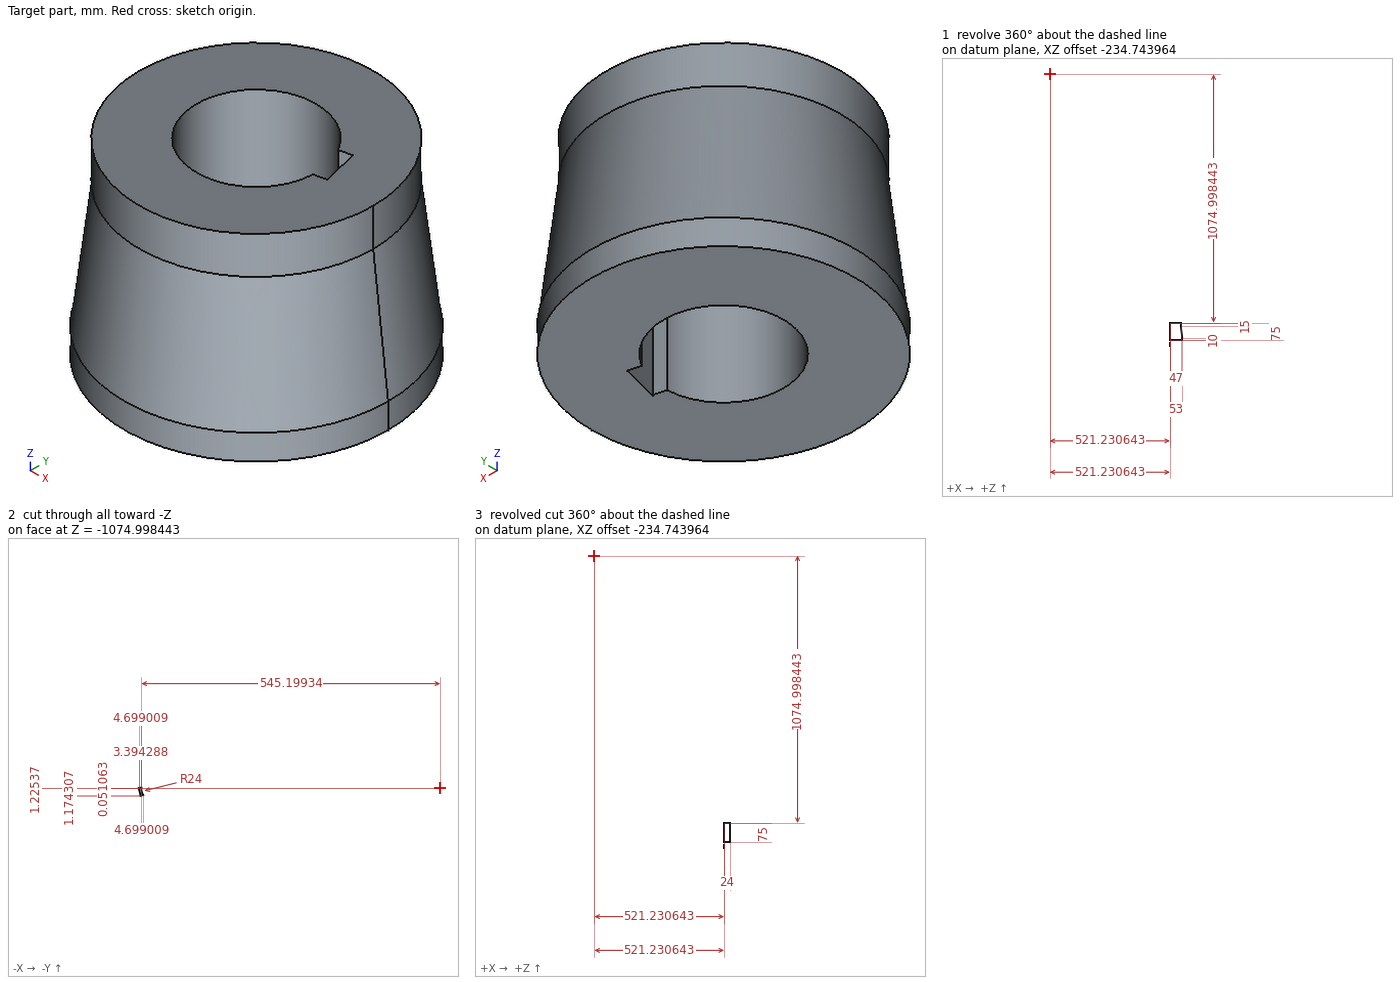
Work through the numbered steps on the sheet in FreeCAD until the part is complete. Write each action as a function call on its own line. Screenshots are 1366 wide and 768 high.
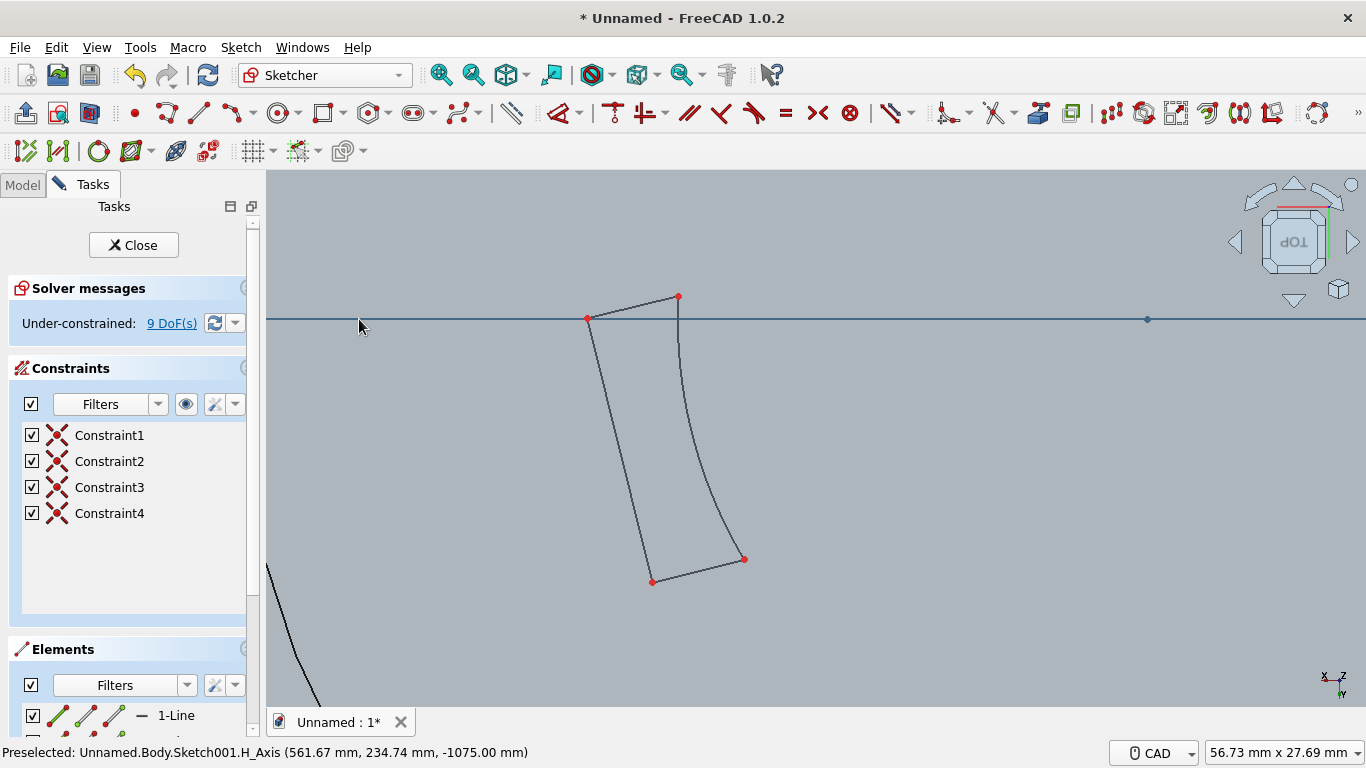
click(614, 114)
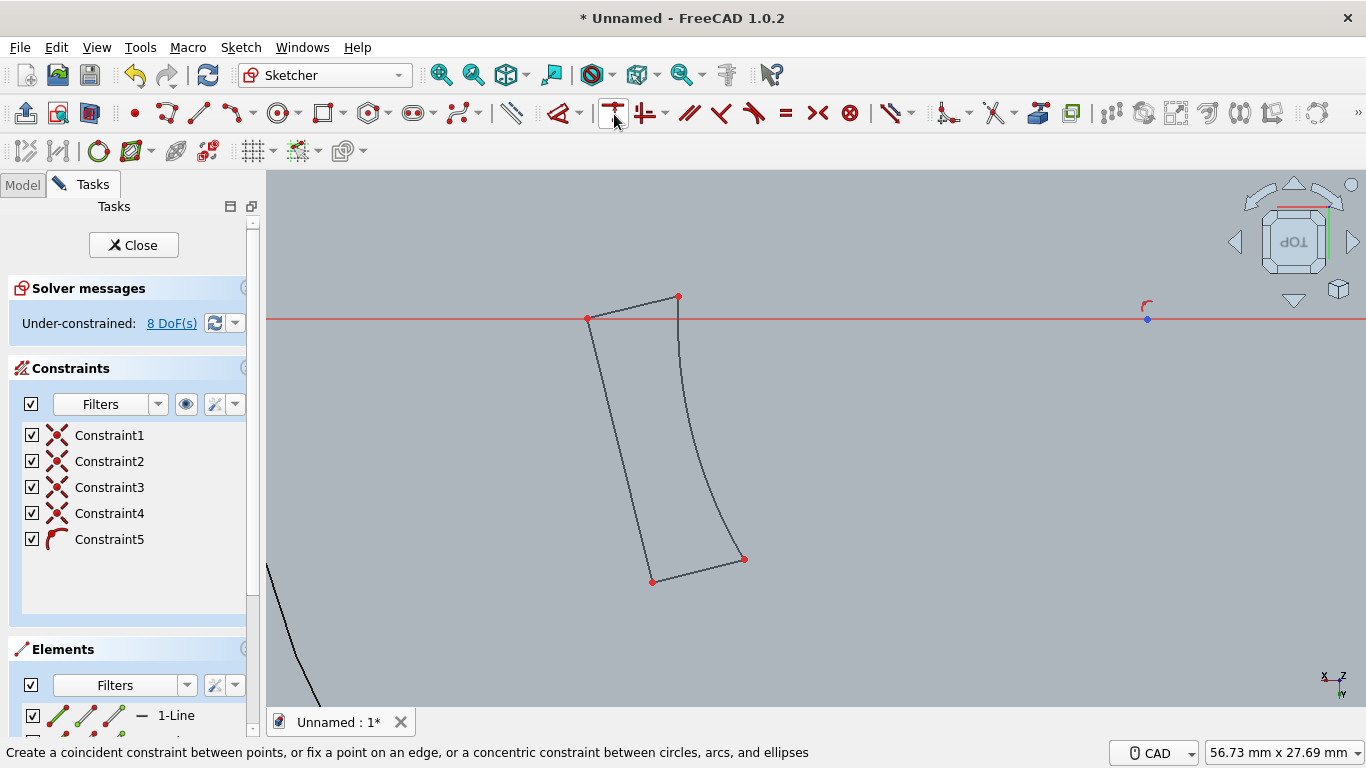
click(558, 114)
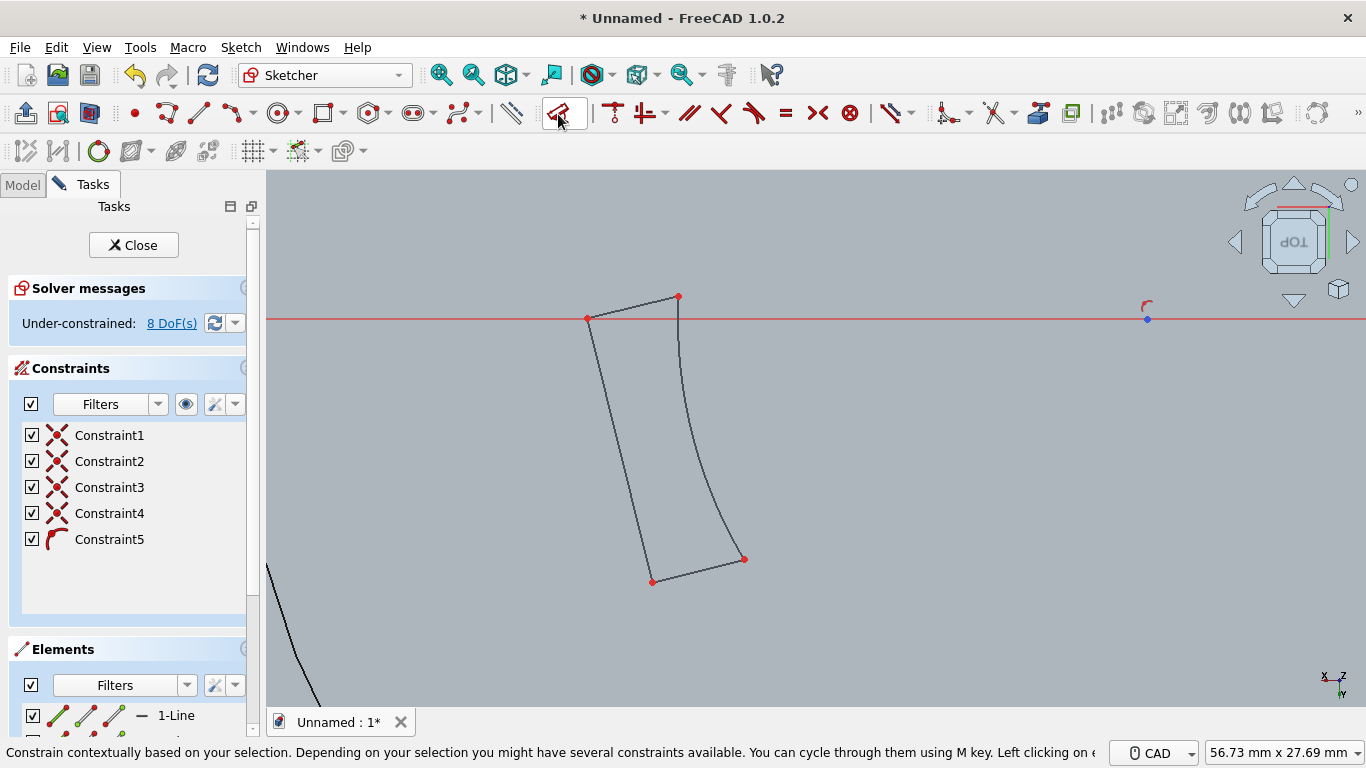
click(682, 379)
click(650, 383)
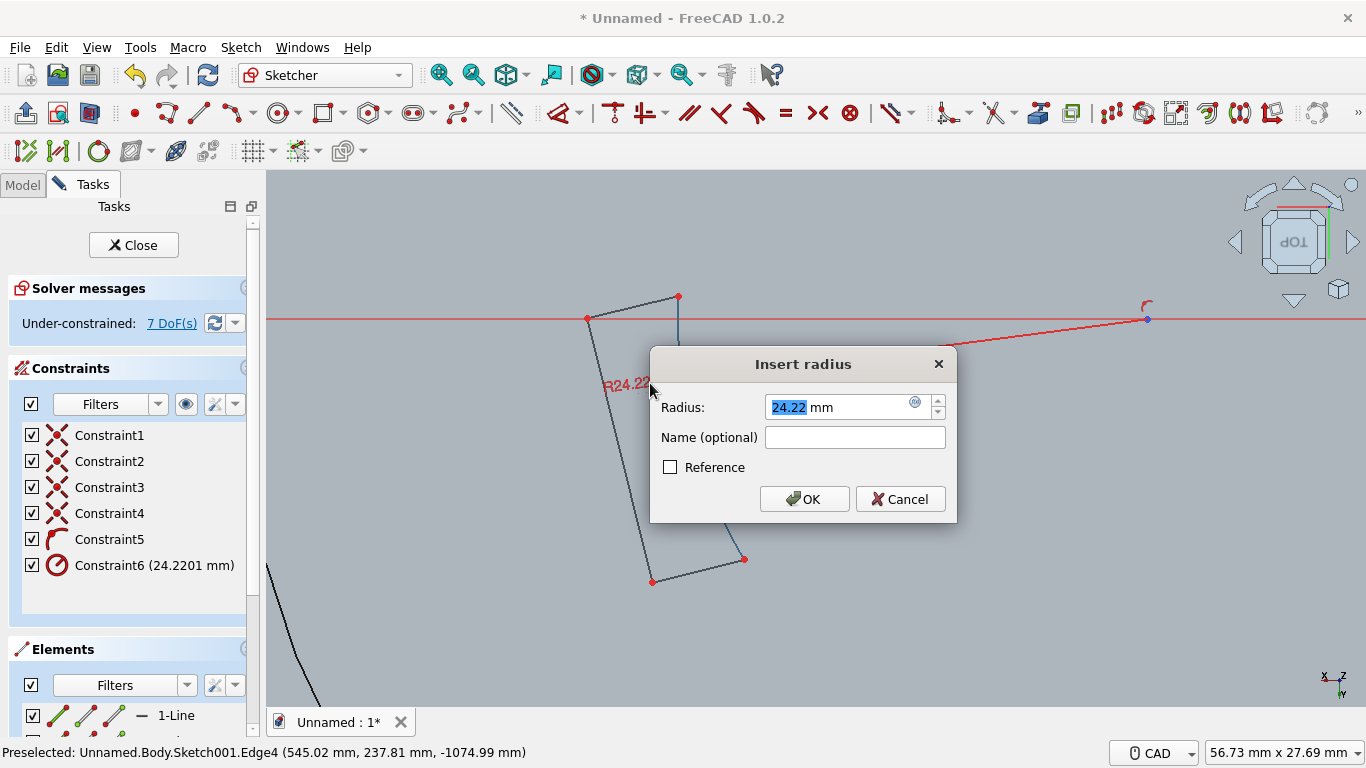
text(24)
key(Return)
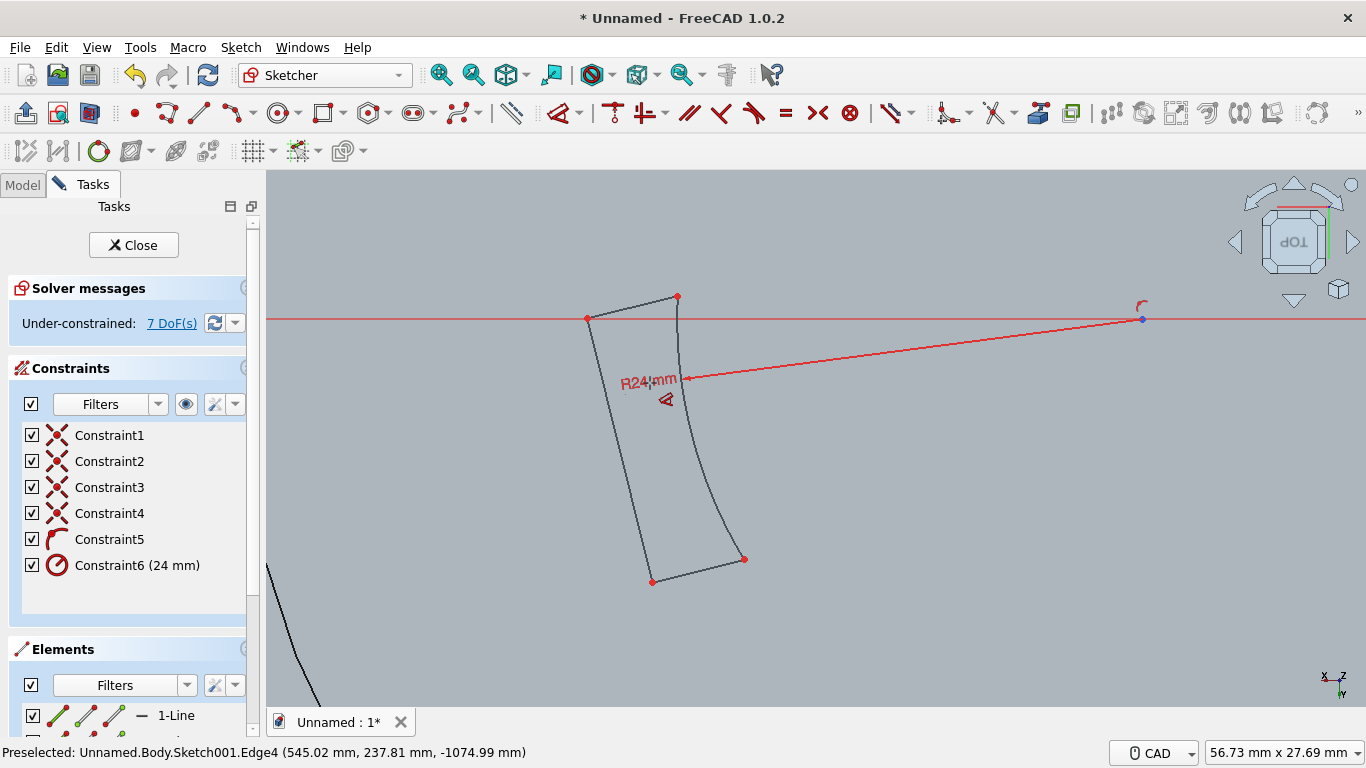
scroll(678, 296, up, 3)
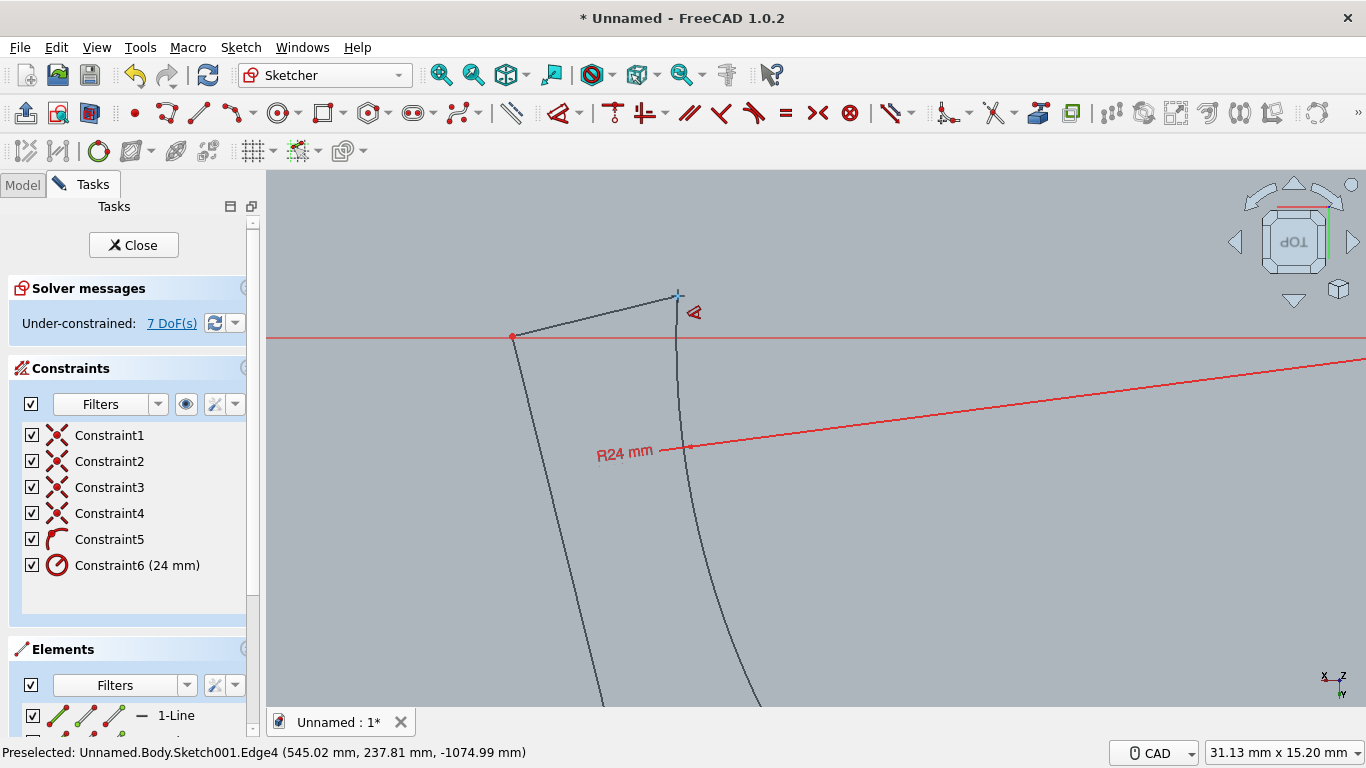
click(677, 296)
click(595, 302)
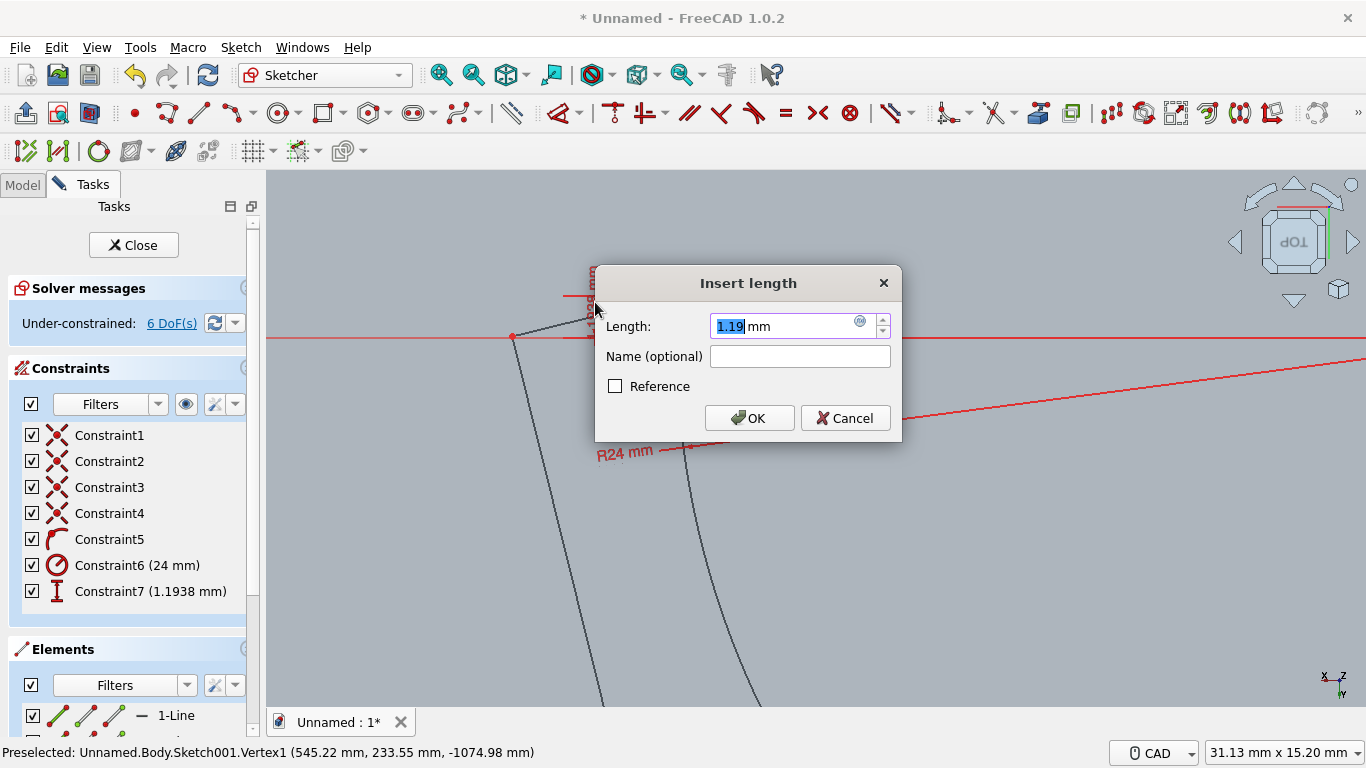
text(1.22537)
key(Return)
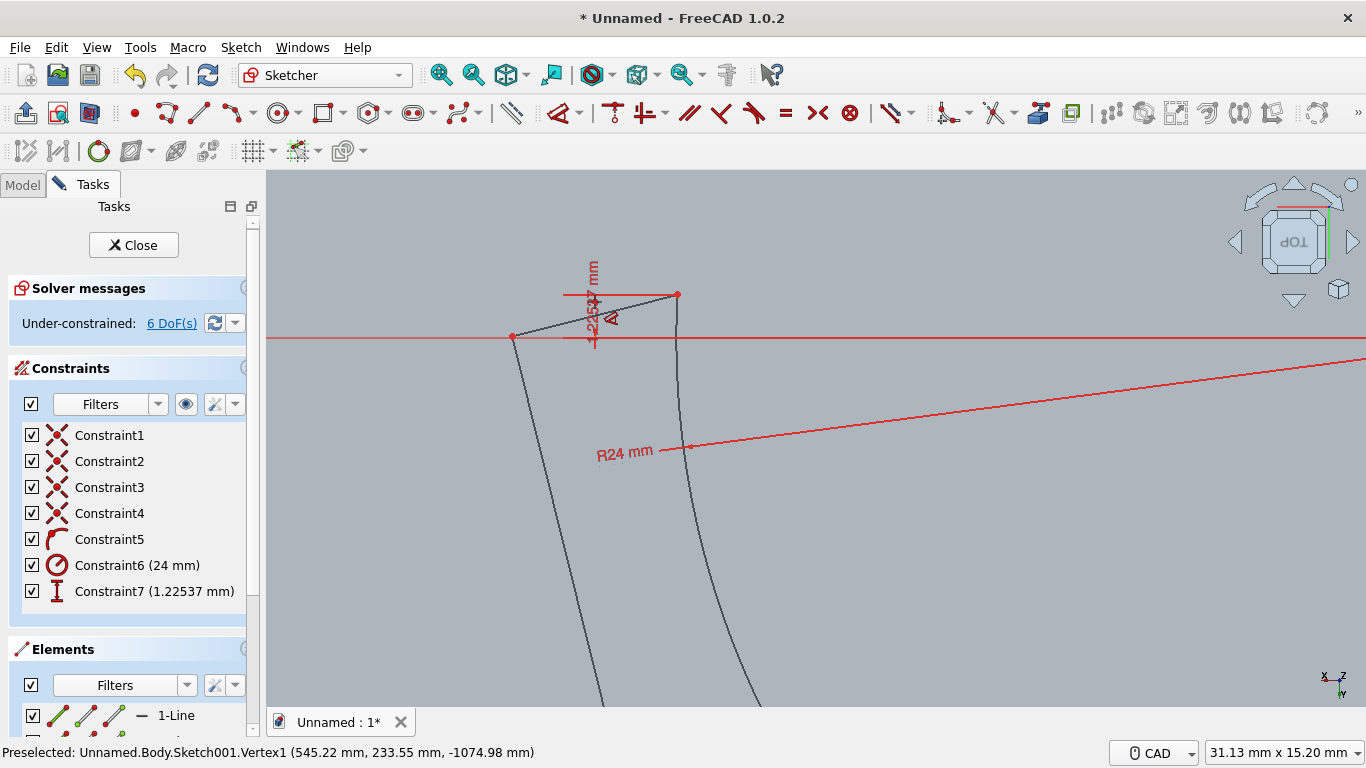
scroll(512, 337, up, 16)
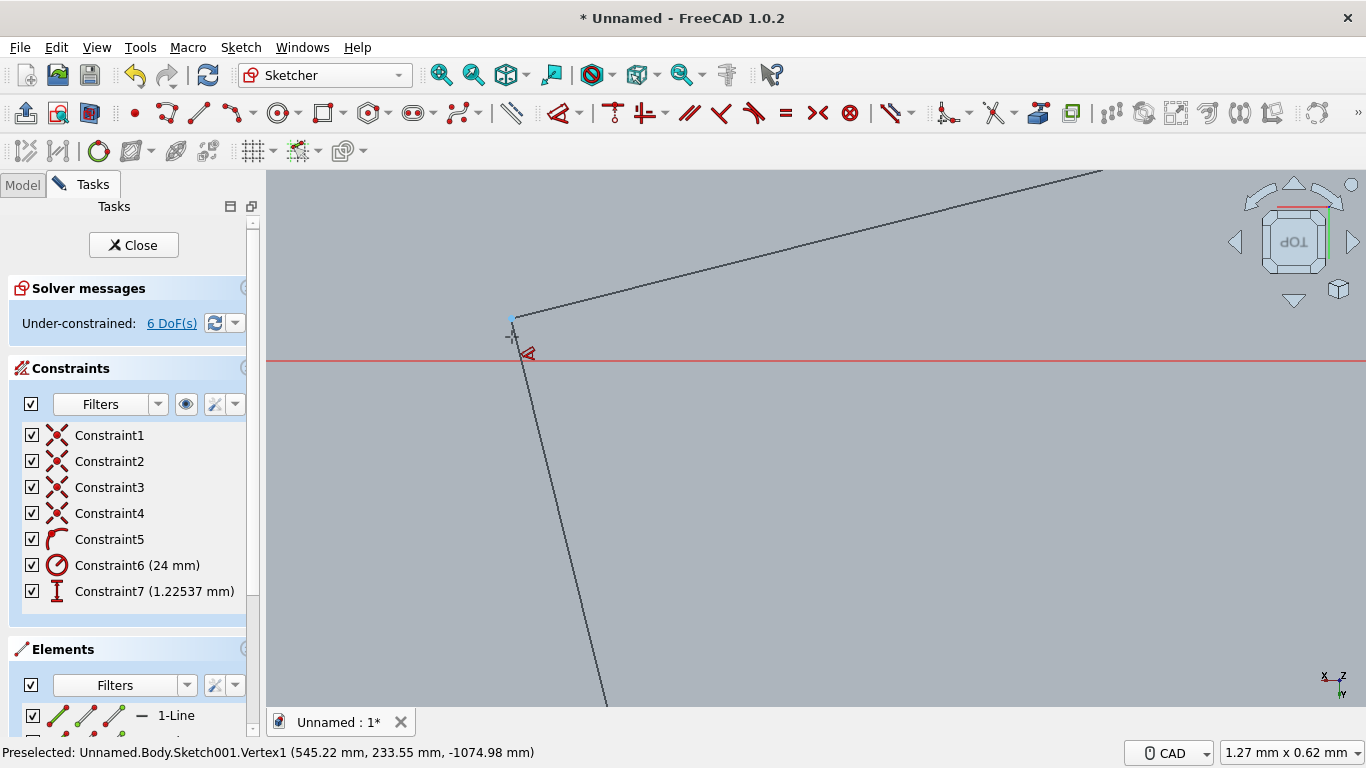
click(511, 319)
click(477, 340)